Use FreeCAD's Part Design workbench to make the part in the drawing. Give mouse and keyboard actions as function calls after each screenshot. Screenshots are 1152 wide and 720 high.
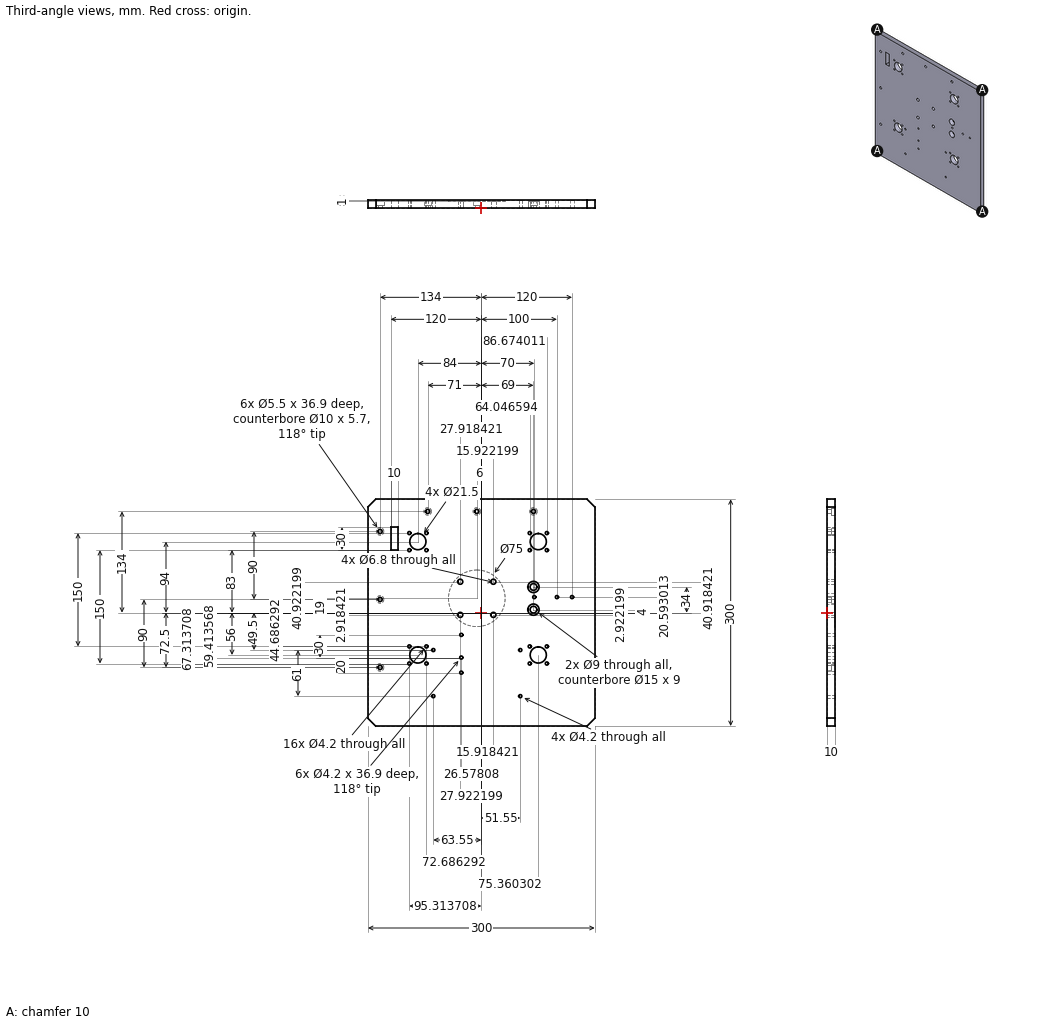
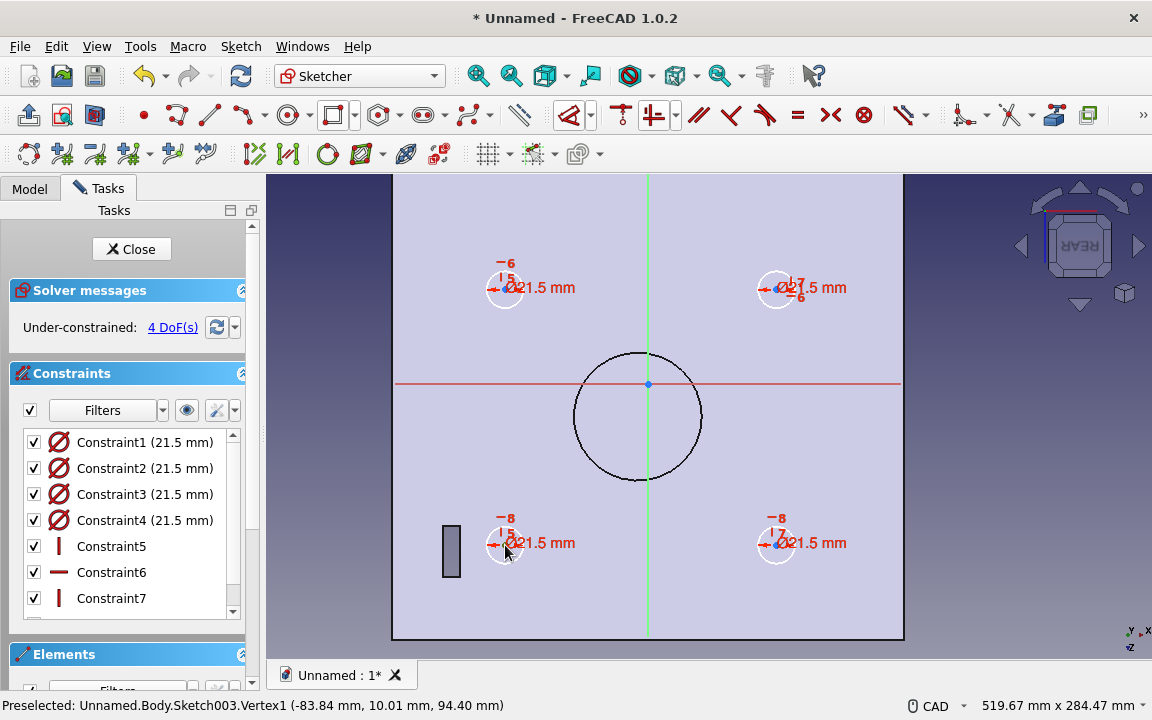
key(l)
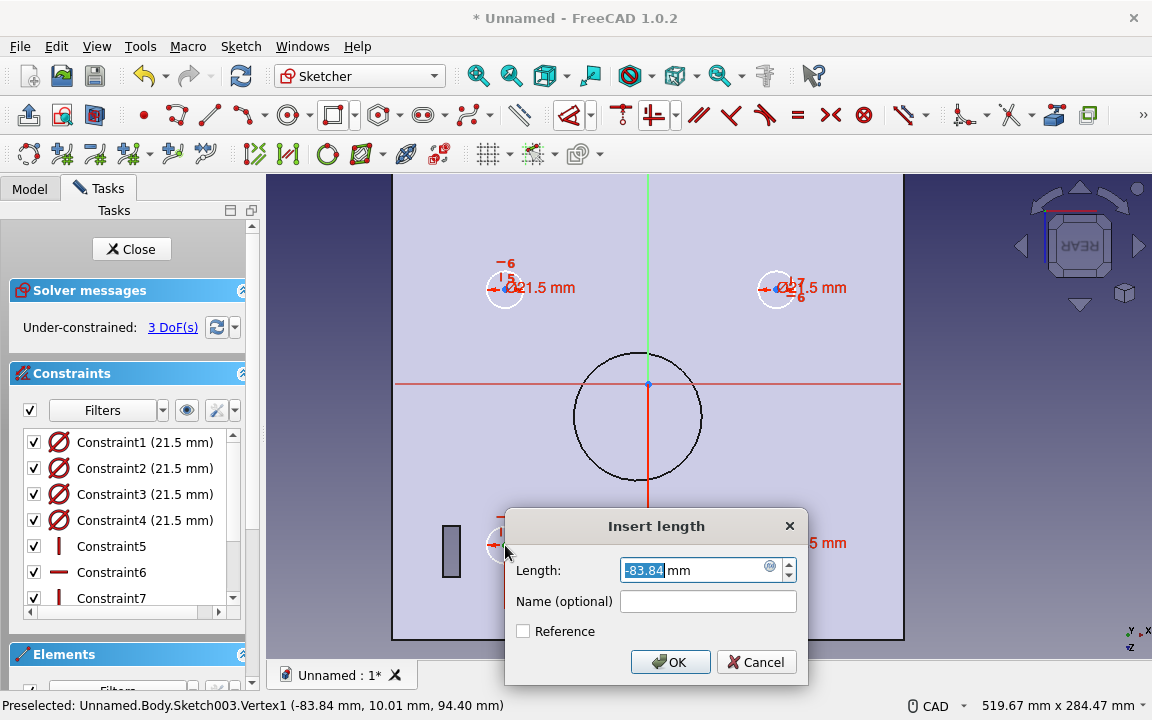
text(-84)
key(Return)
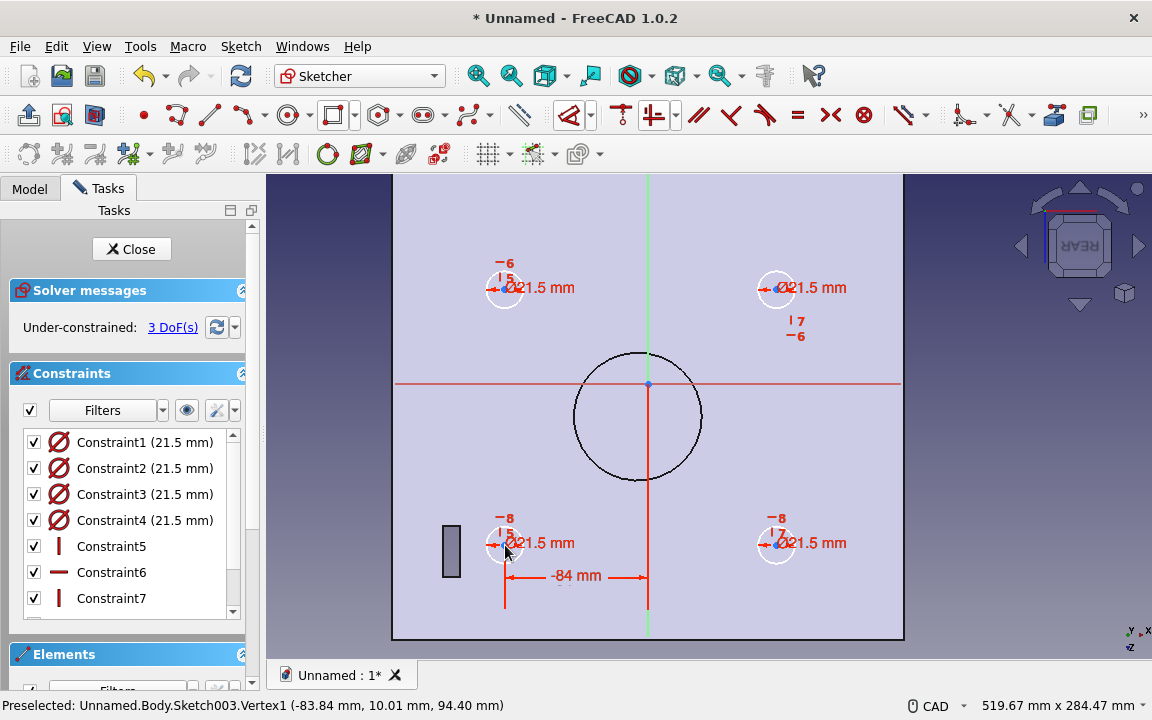
click(505, 545)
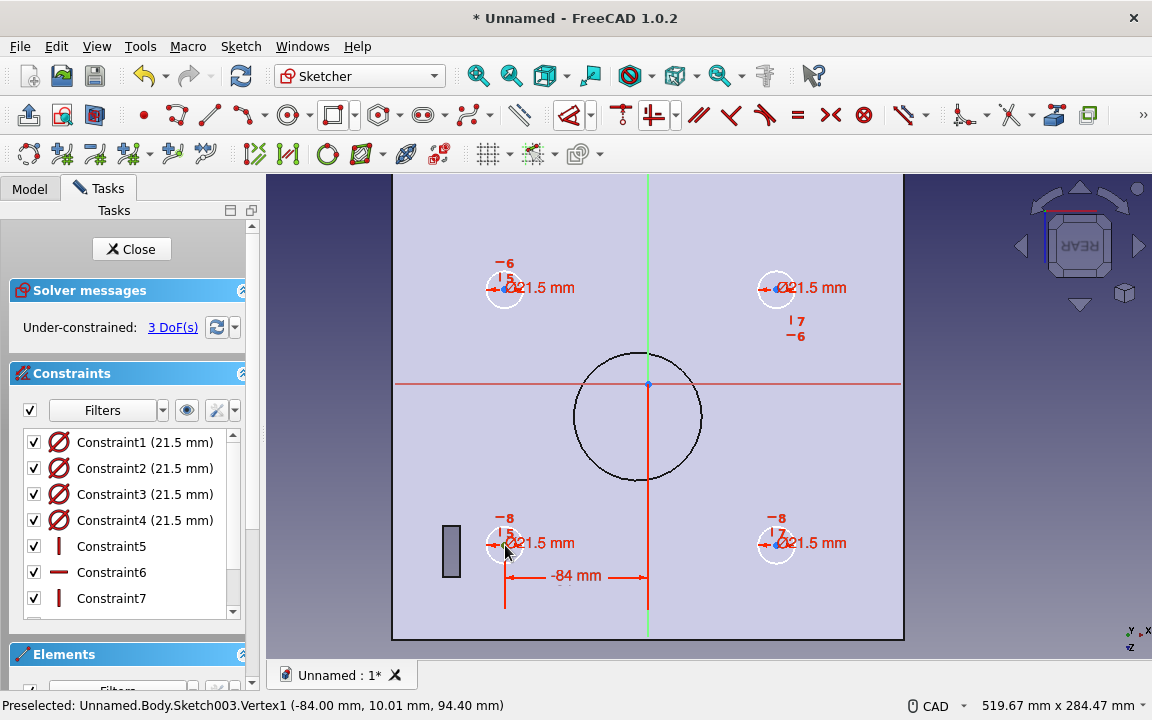
click(590, 116)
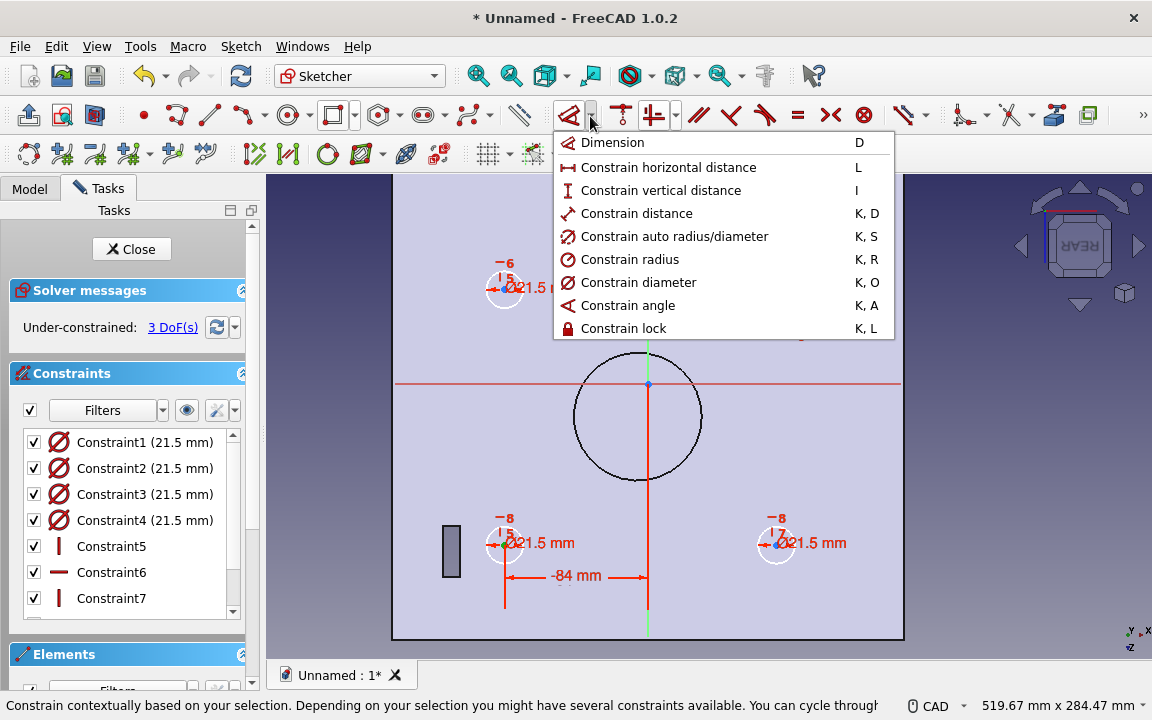
click(724, 190)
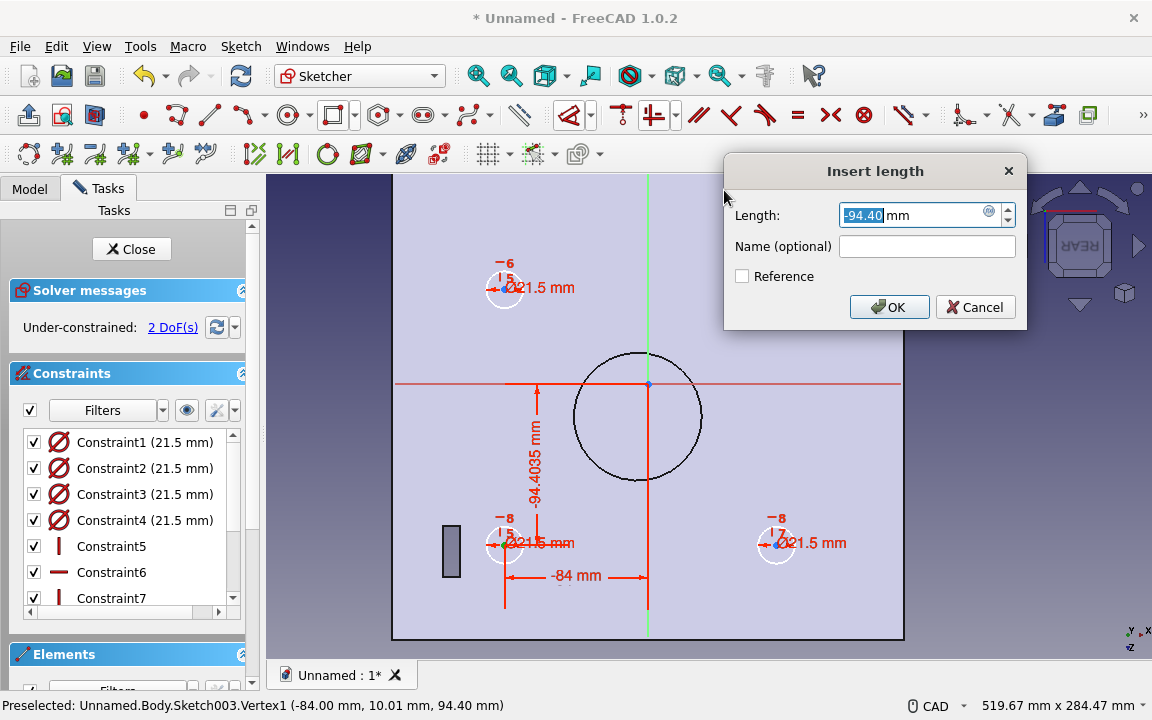
text(-94)
key(Return)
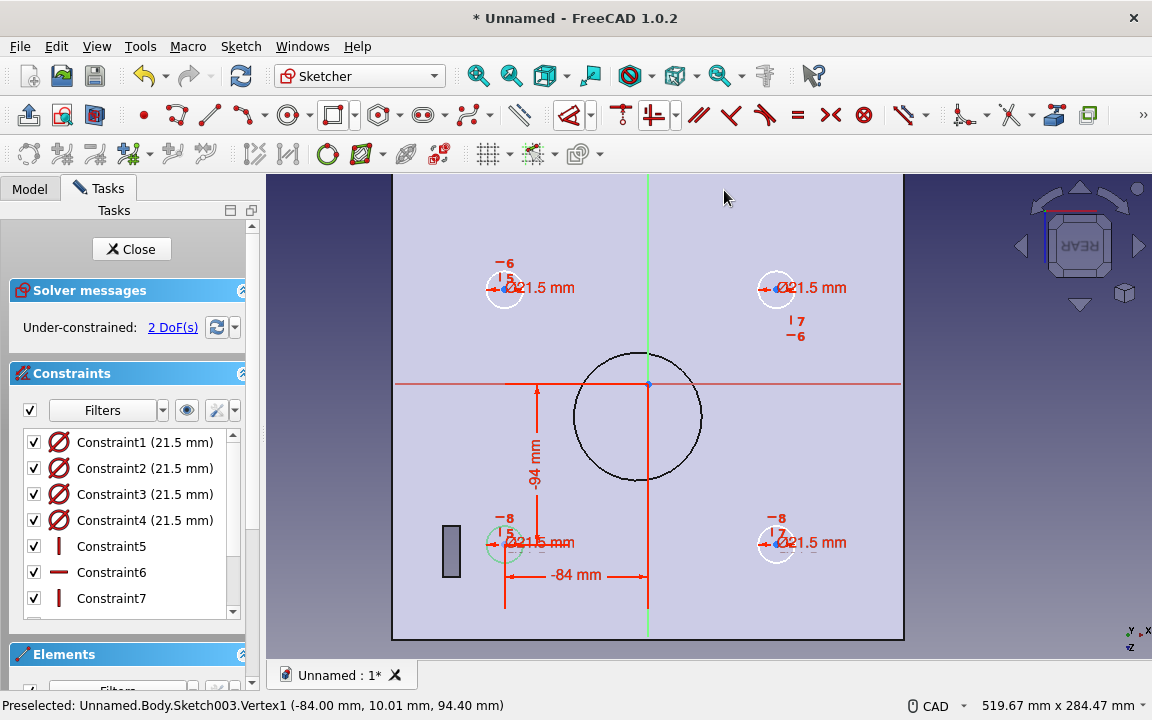
click(505, 290)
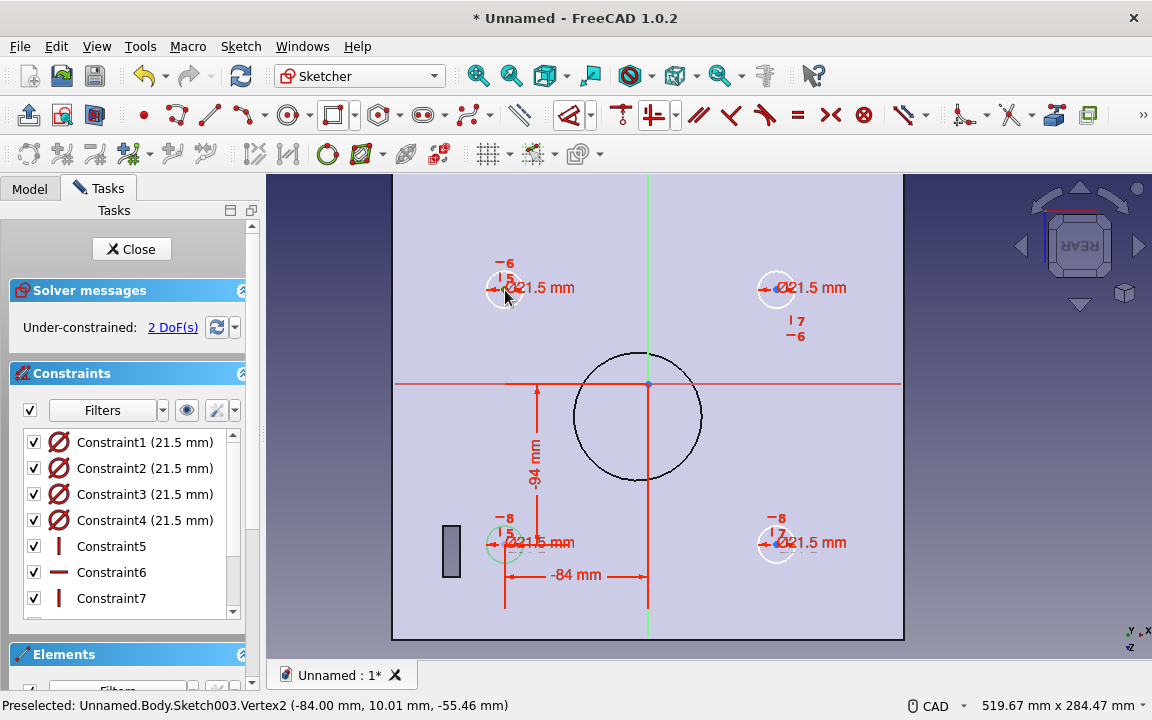
key(i)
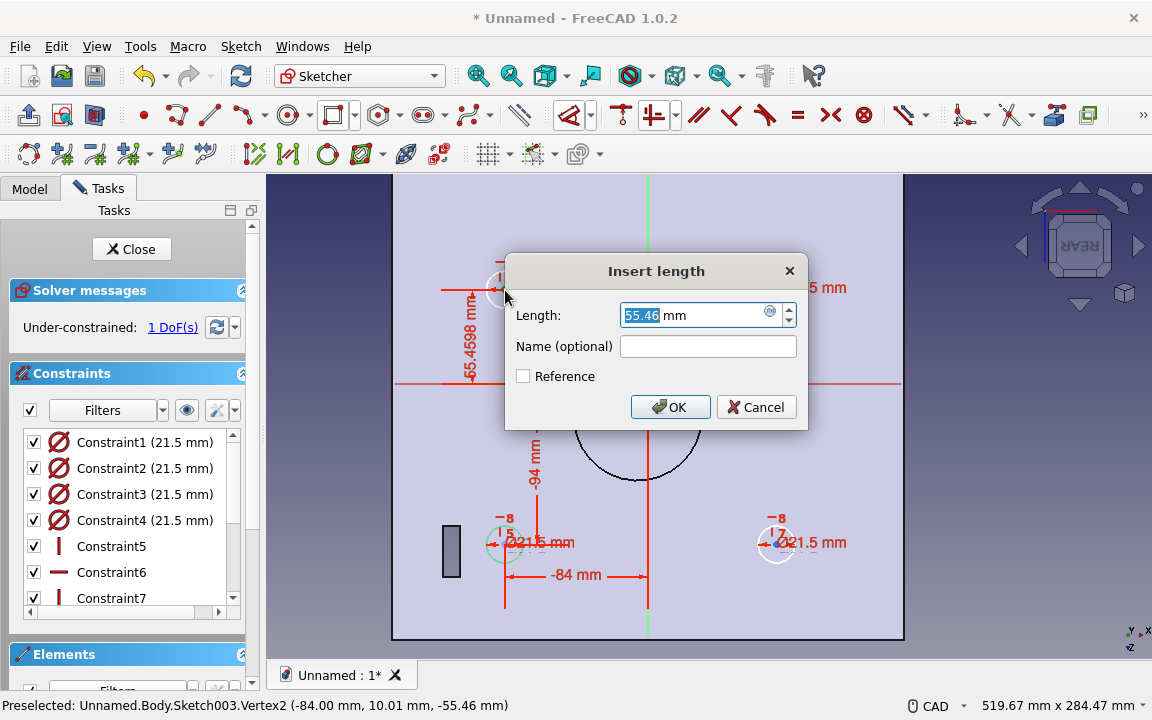
text(56)
key(Return)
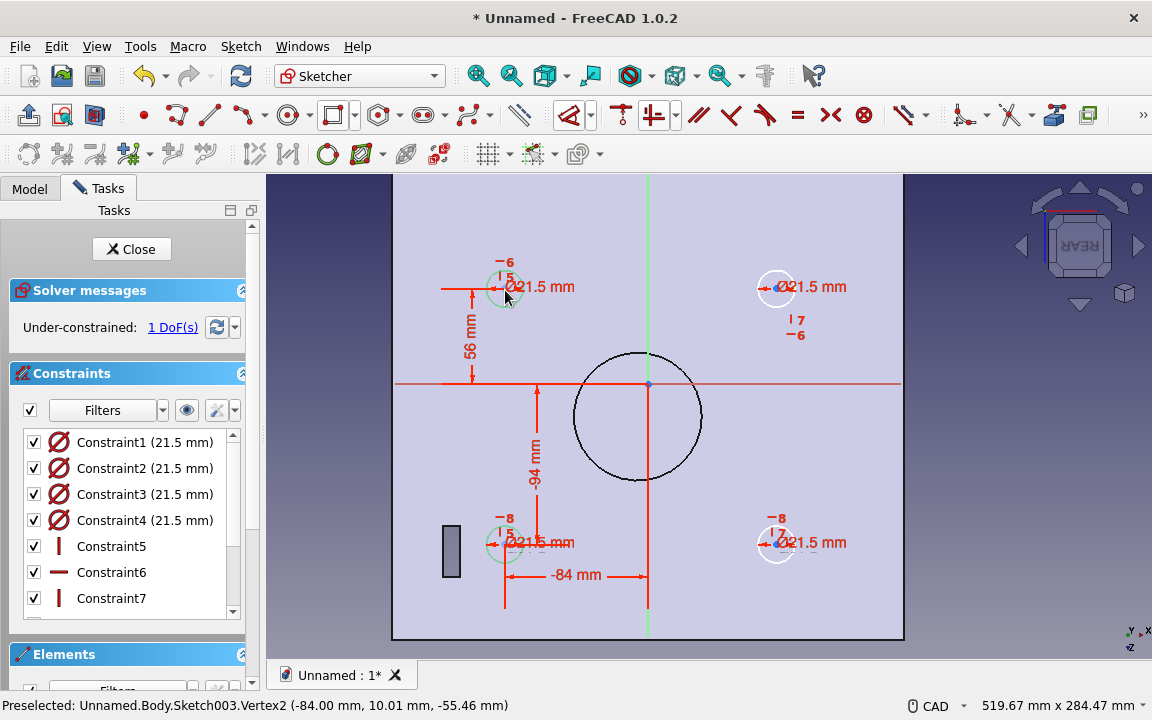
click(777, 289)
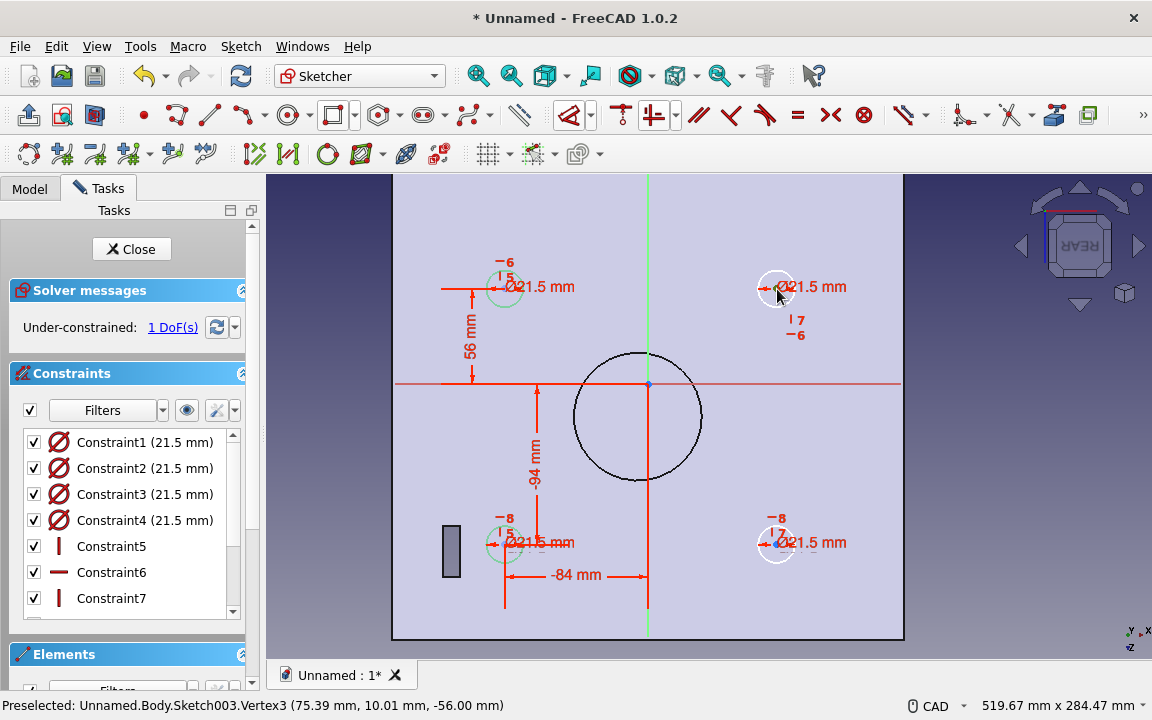
key(l)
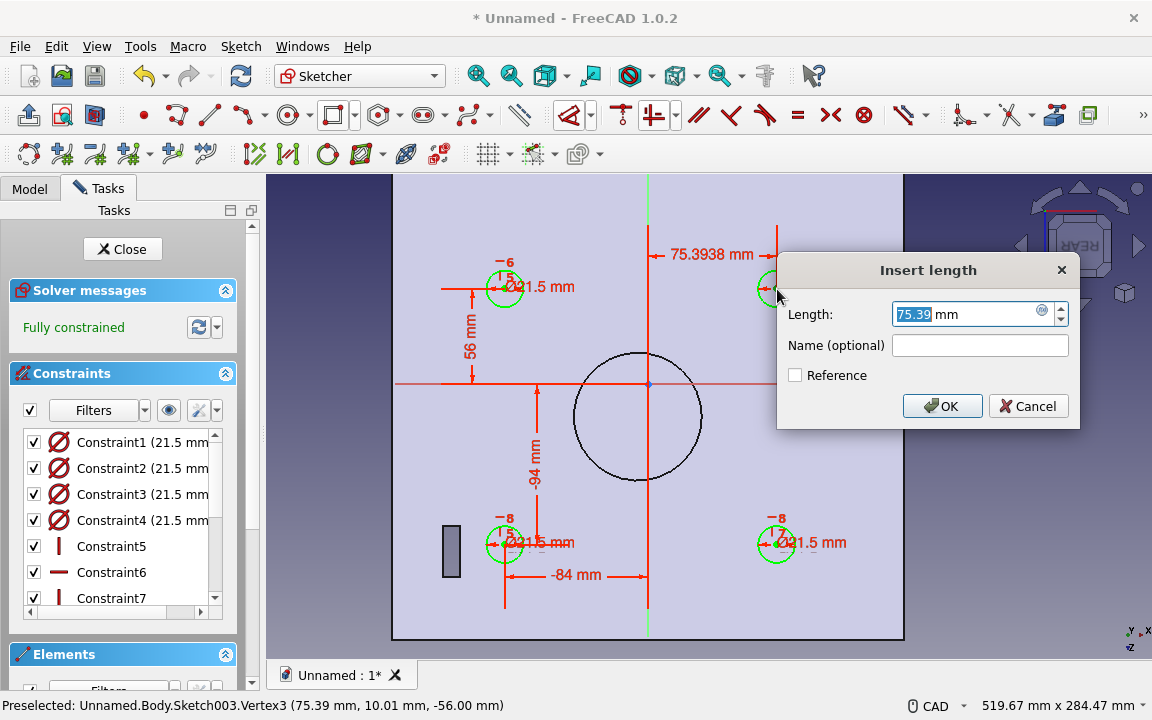
text(75.360302)
key(Return)